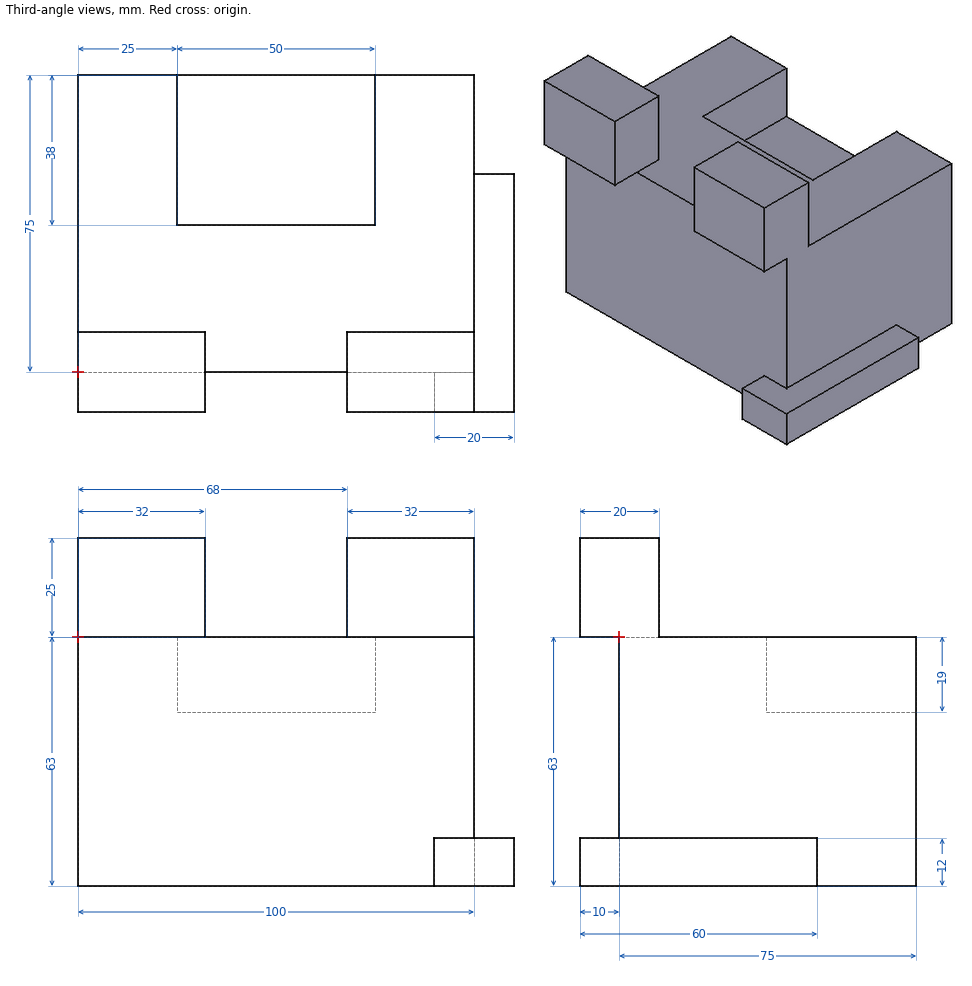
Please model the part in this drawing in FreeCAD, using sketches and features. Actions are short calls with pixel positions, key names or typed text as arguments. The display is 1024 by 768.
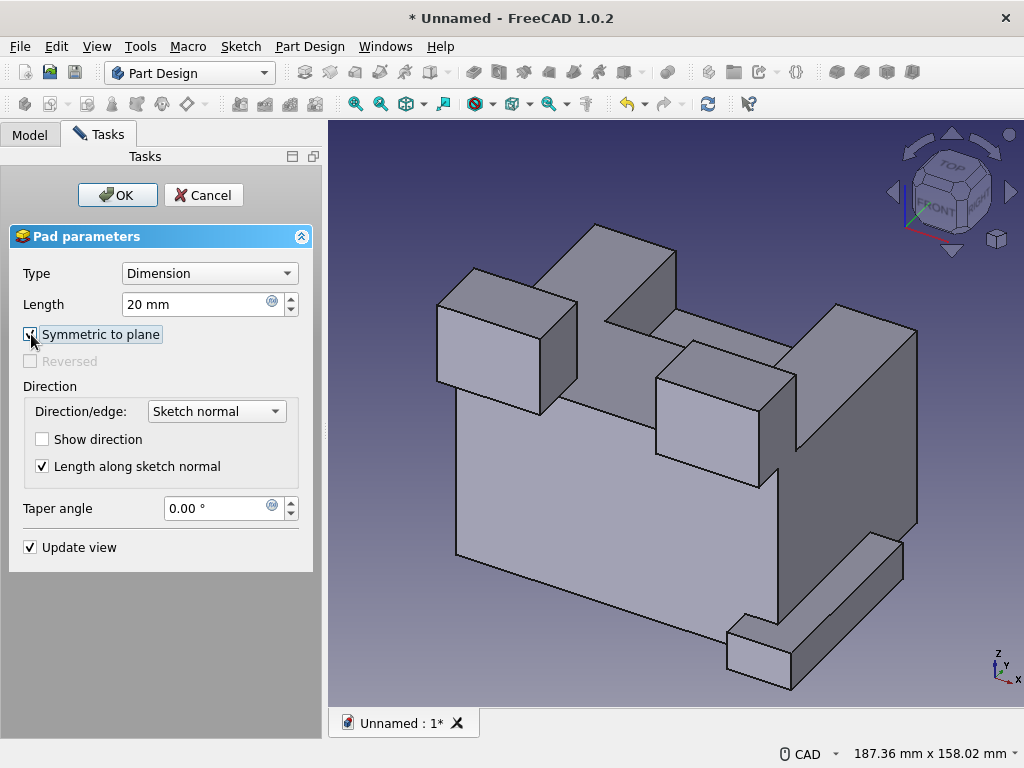
click(118, 195)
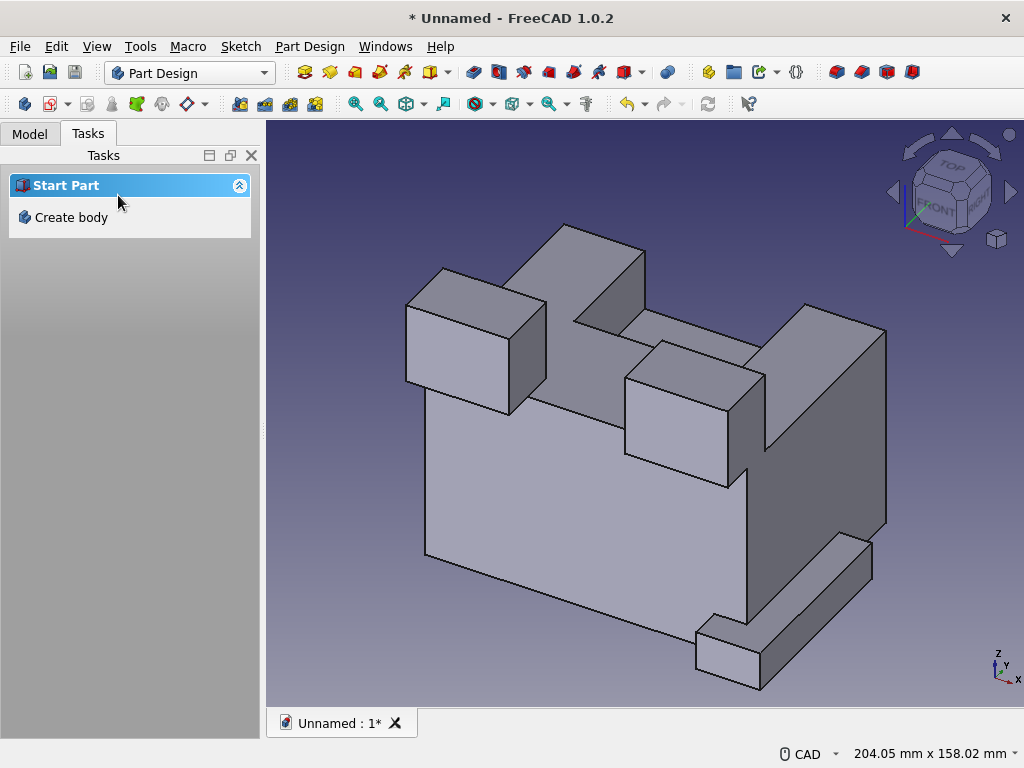
key(0)